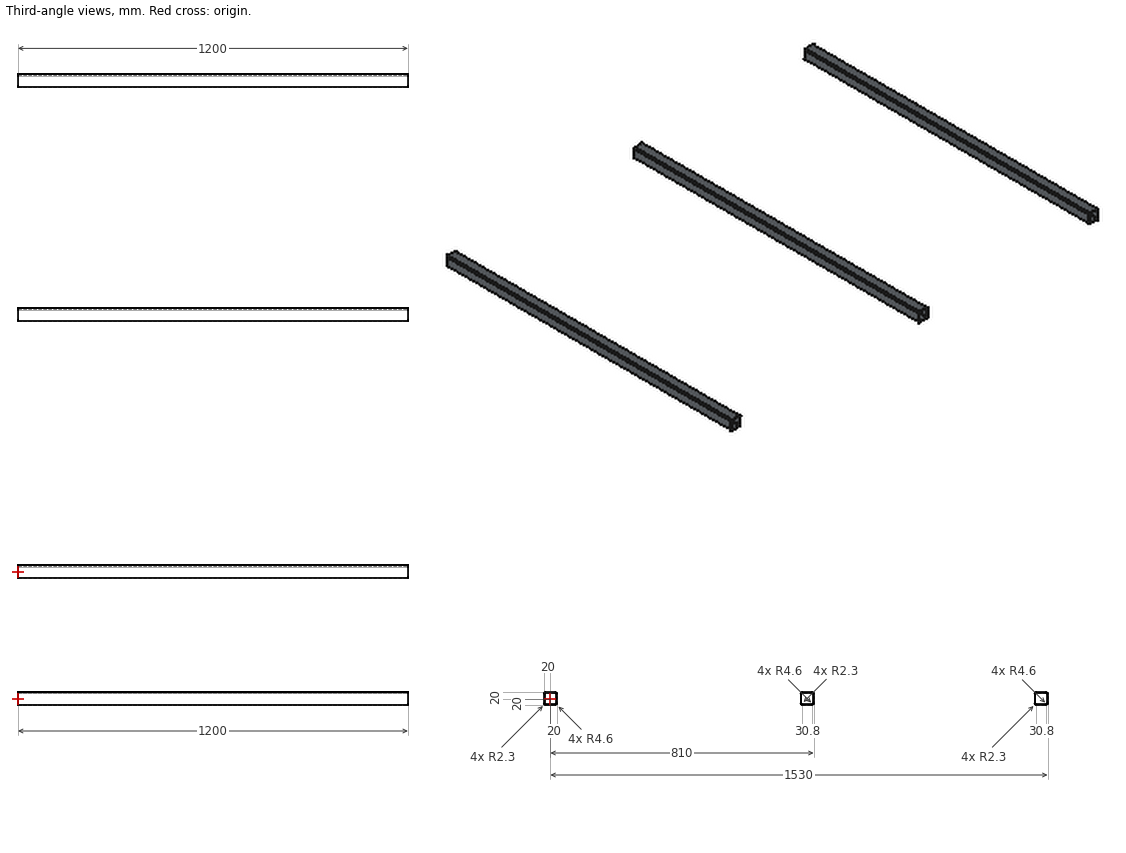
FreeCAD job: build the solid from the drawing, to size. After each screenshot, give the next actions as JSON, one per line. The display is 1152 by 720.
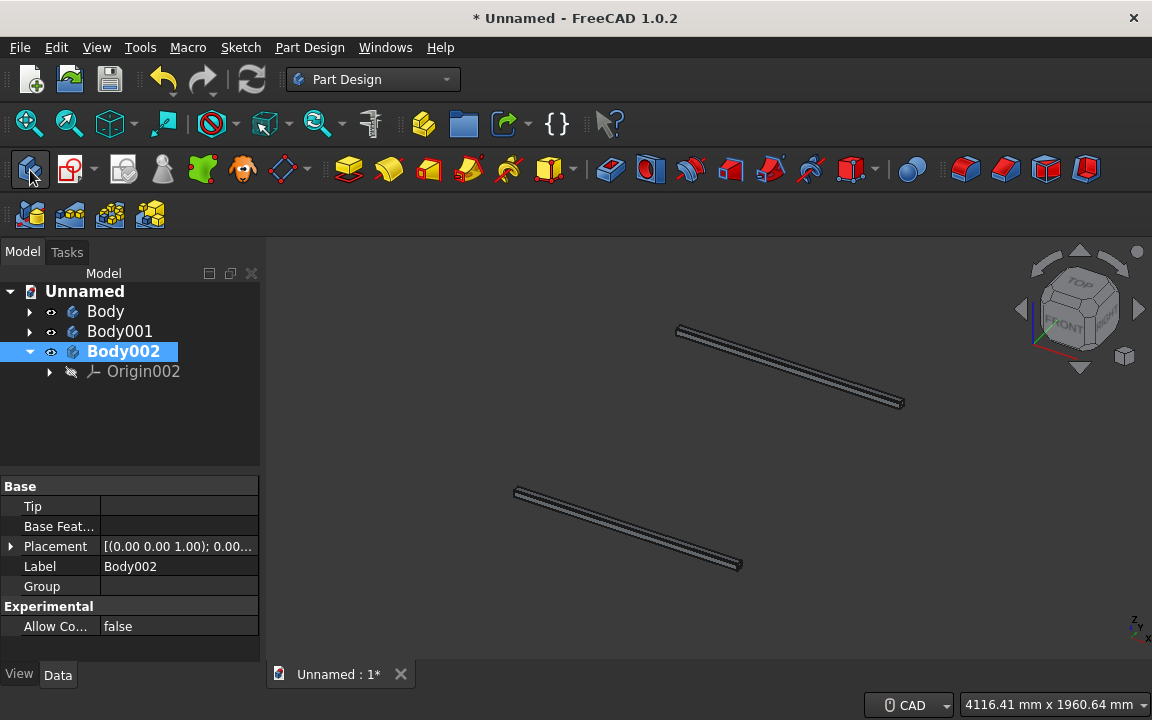
{"action": "left_click", "coordinate": [306, 619]}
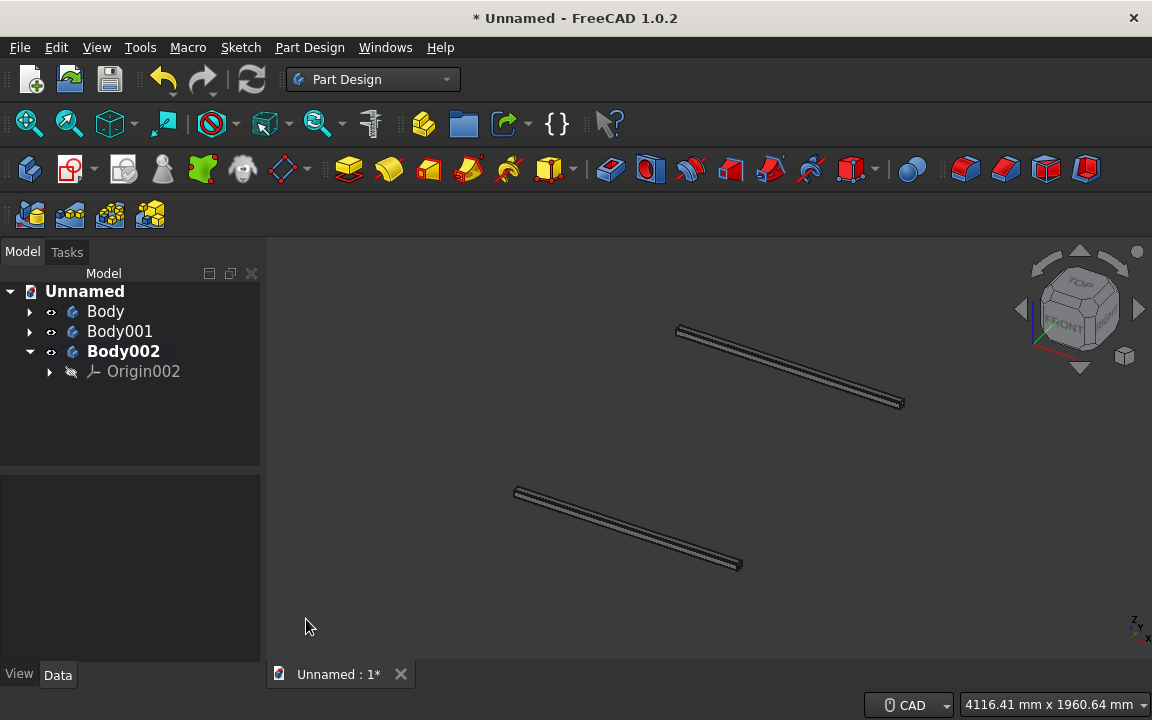
{"action": "left_click", "coordinate": [70, 170]}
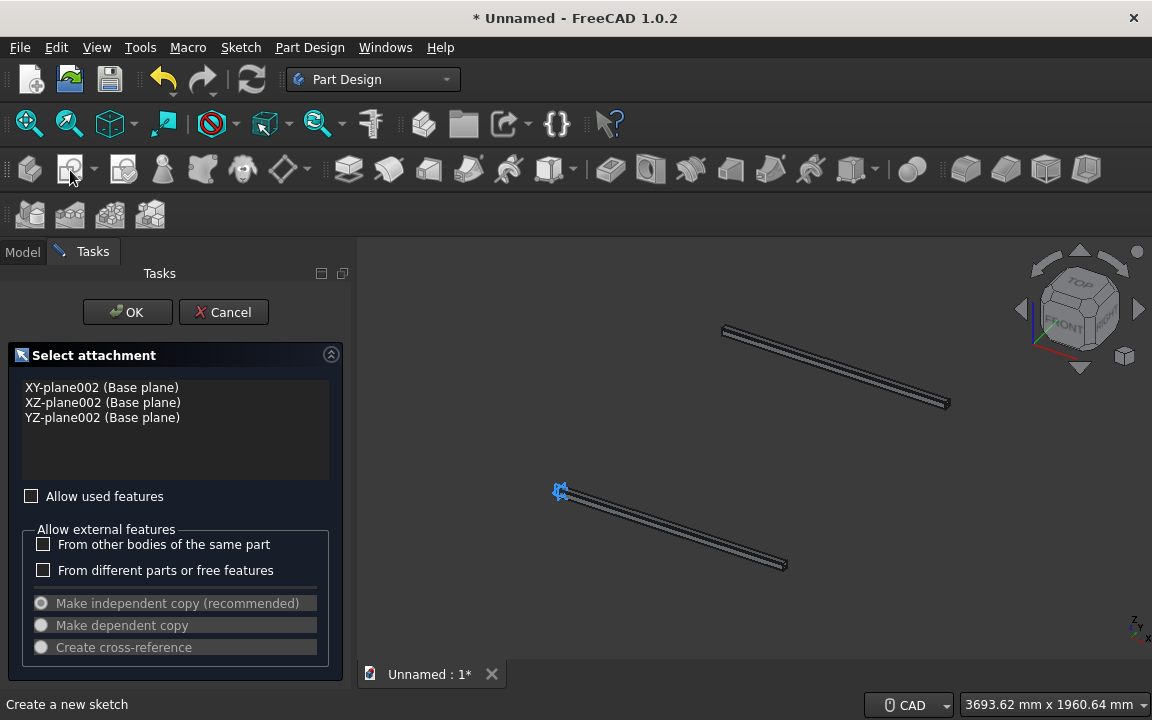
{"action": "left_click", "coordinate": [82, 418]}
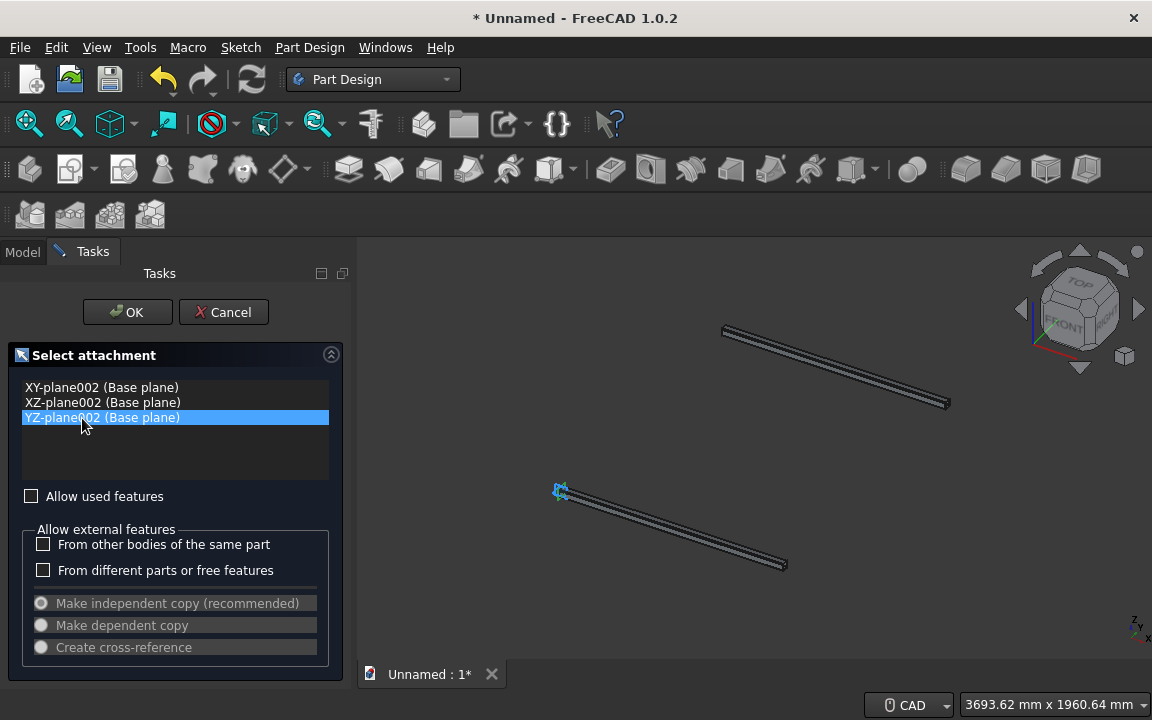
{"action": "left_click", "coordinate": [128, 312]}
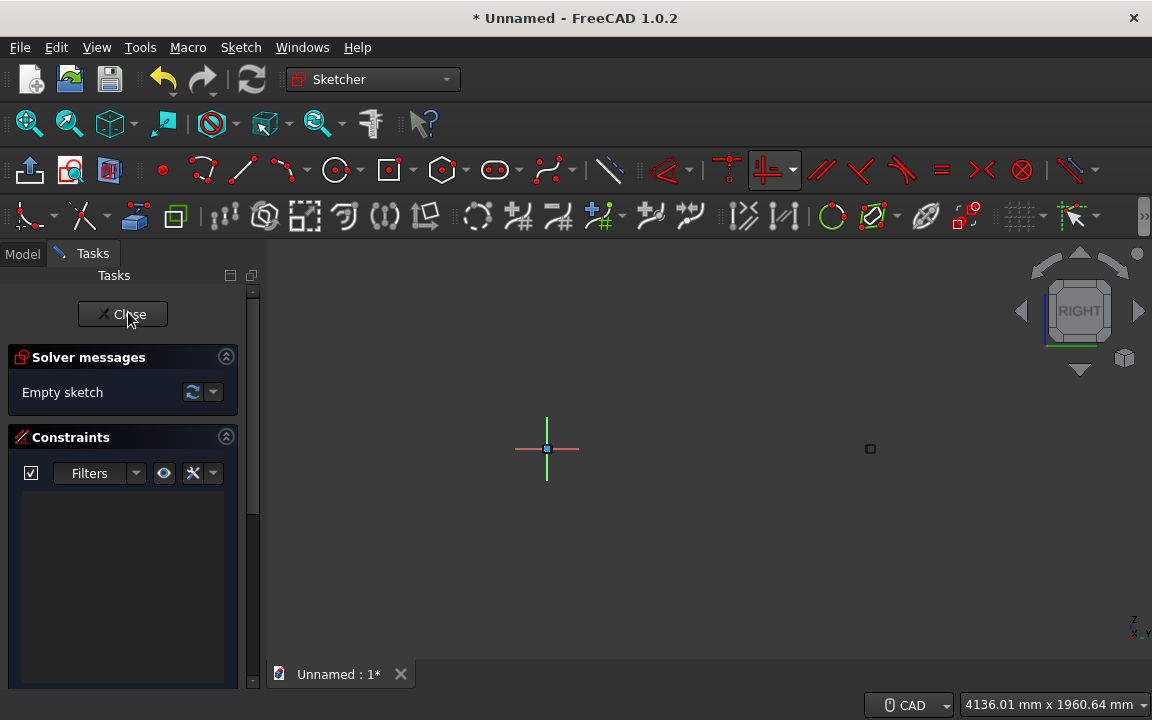
{"action": "scroll", "coordinate": [720, 449], "scroll_direction": "up", "scroll_amount": 15}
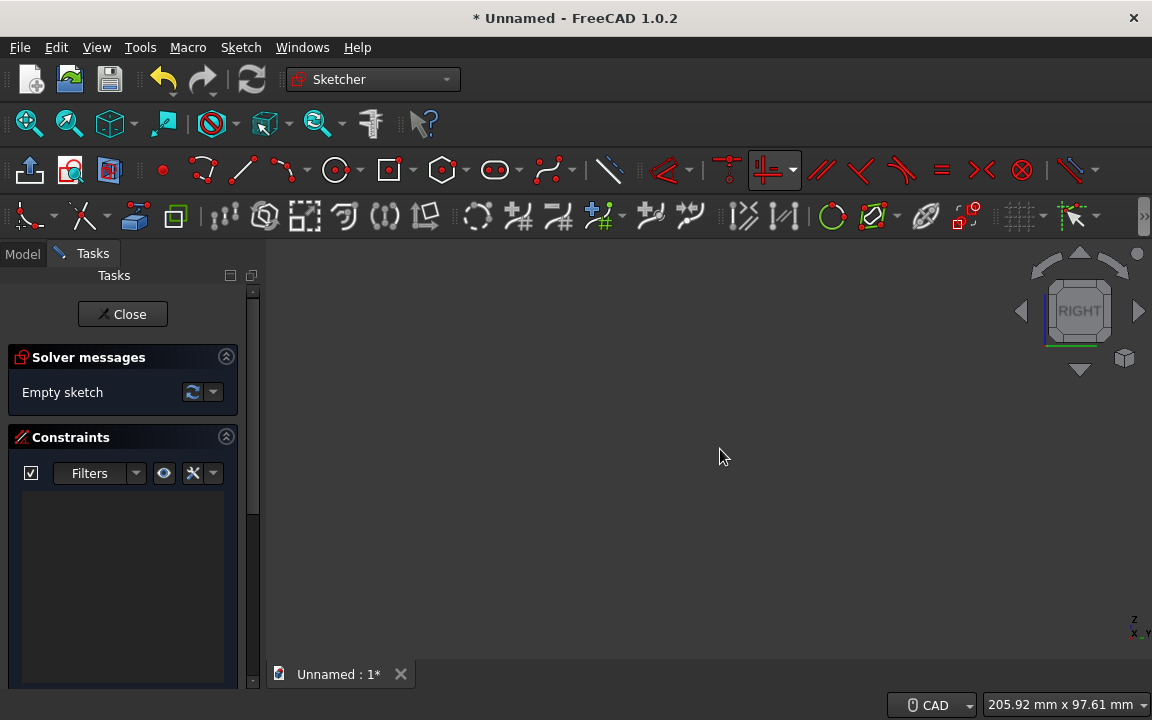
{"action": "scroll", "coordinate": [639, 420], "scroll_direction": "up", "scroll_amount": 2}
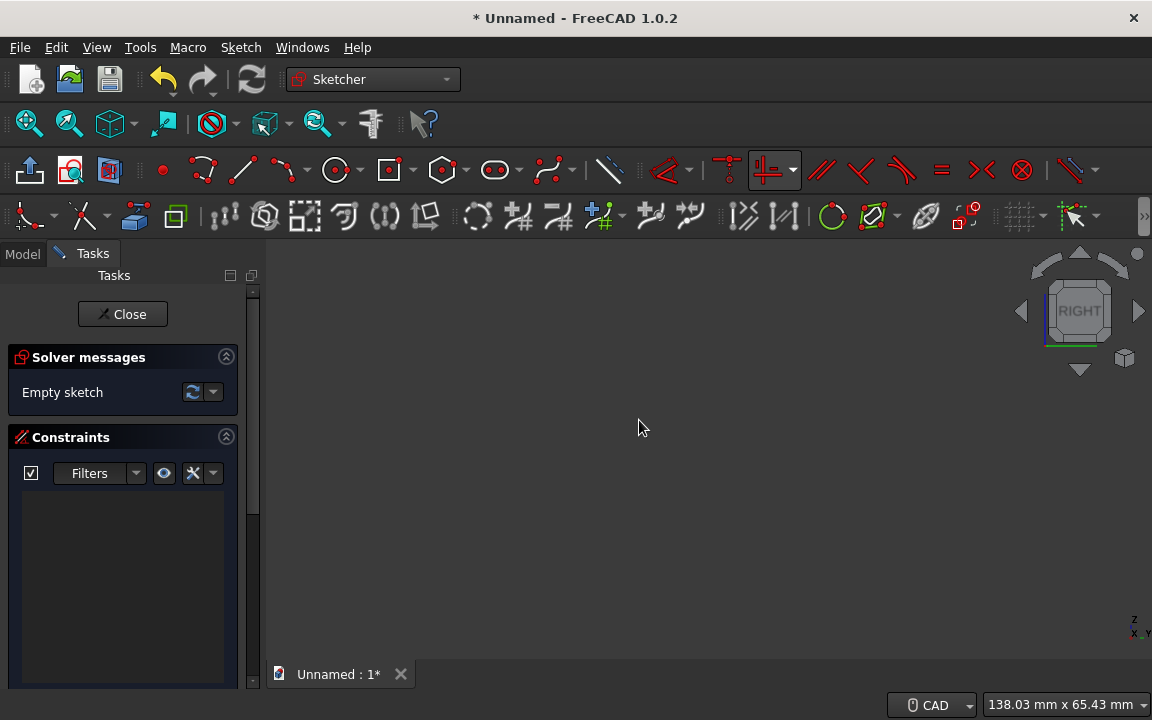
{"action": "left_click", "coordinate": [244, 170]}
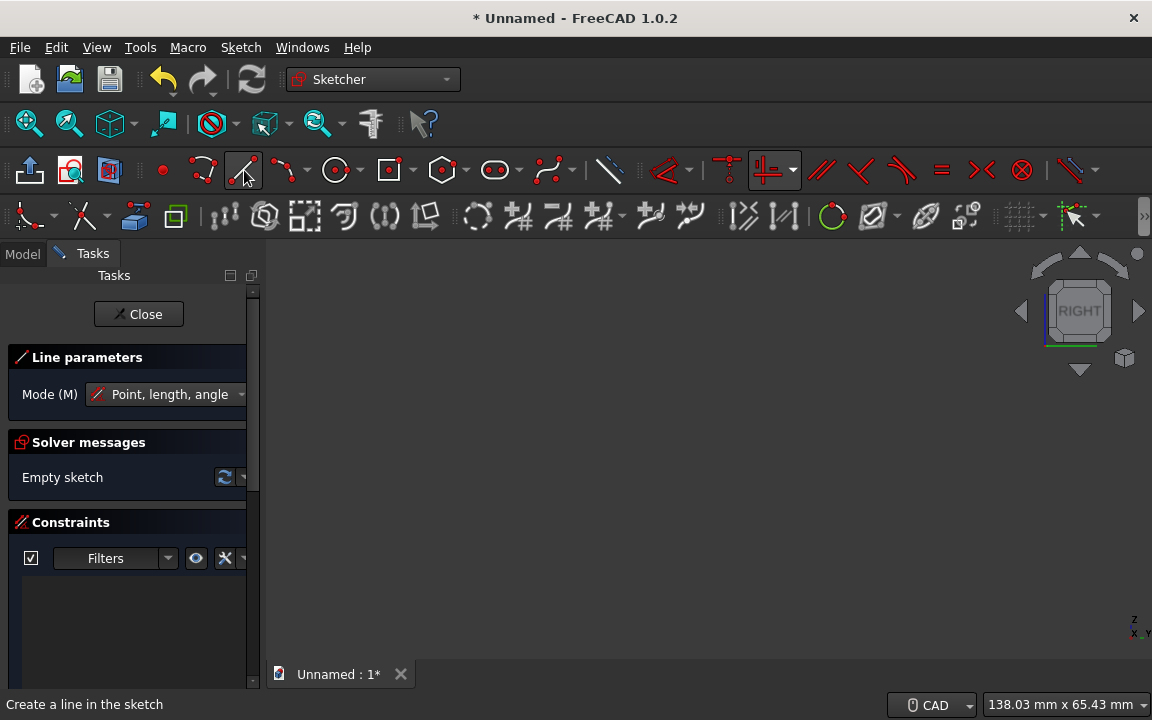
{"action": "left_click", "coordinate": [541, 577]}
{"action": "left_click", "coordinate": [739, 577]}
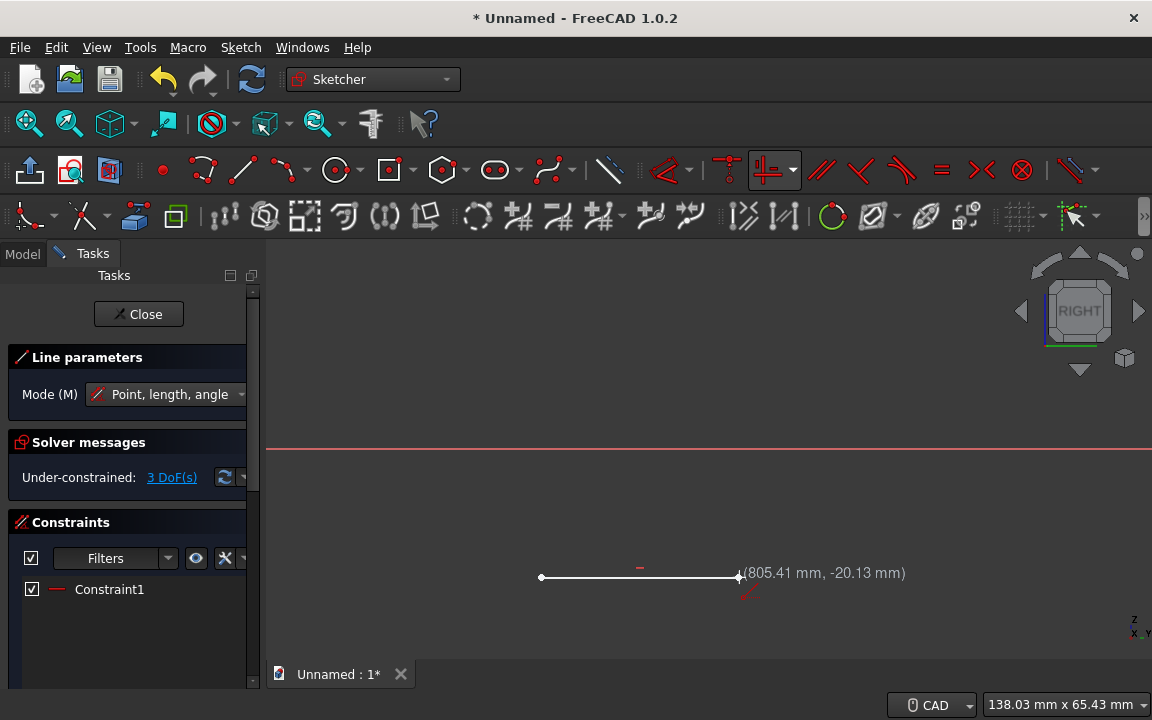
{"action": "left_click", "coordinate": [768, 548]}
{"action": "left_click", "coordinate": [768, 350]}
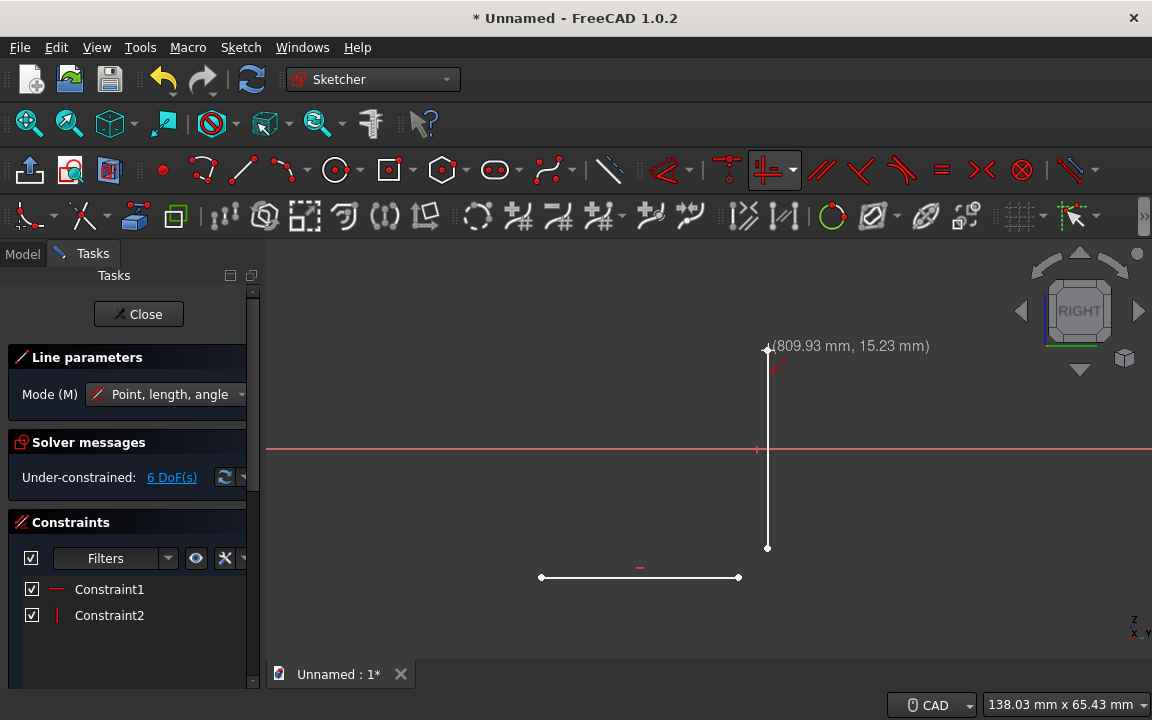
{"action": "left_click", "coordinate": [739, 320]}
{"action": "left_click", "coordinate": [541, 320]}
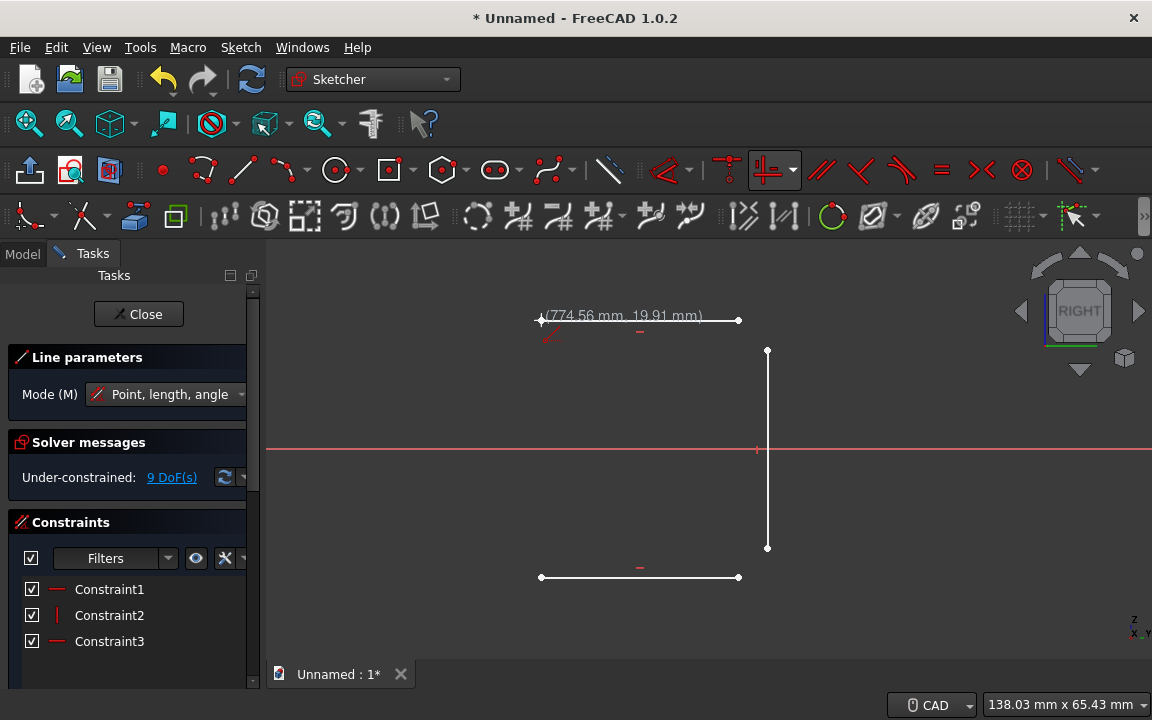
{"action": "left_click", "coordinate": [512, 350]}
{"action": "left_click", "coordinate": [512, 548]}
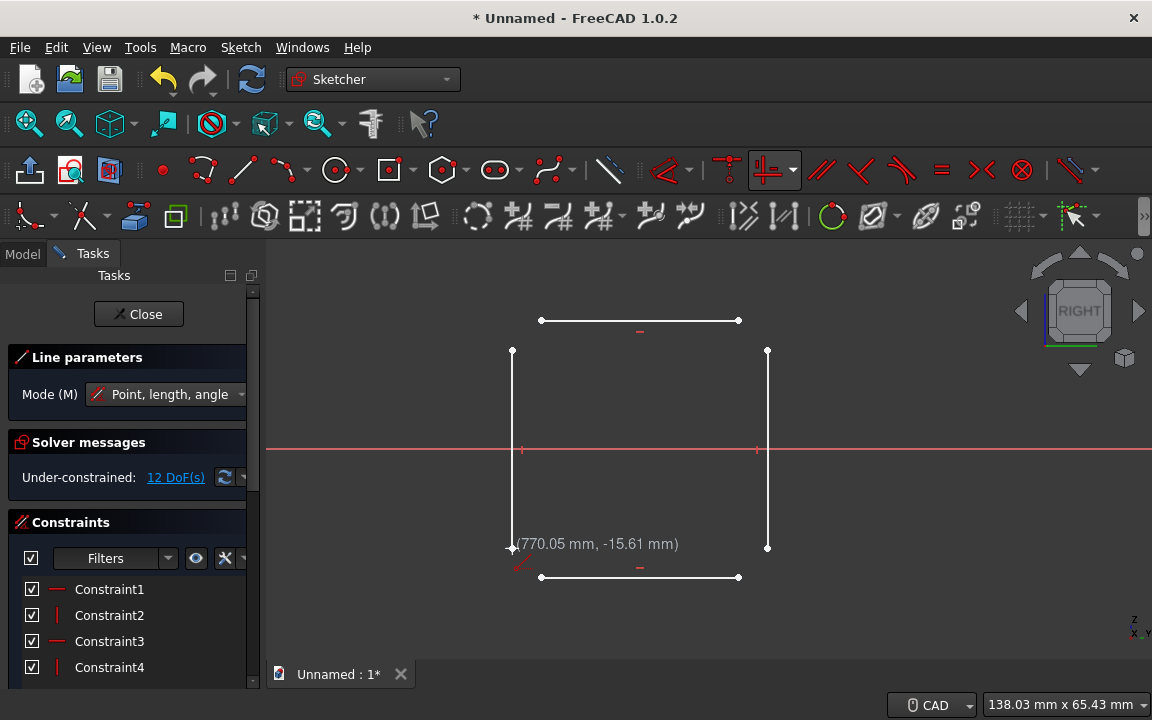
{"action": "key", "text": "g 3 a"}